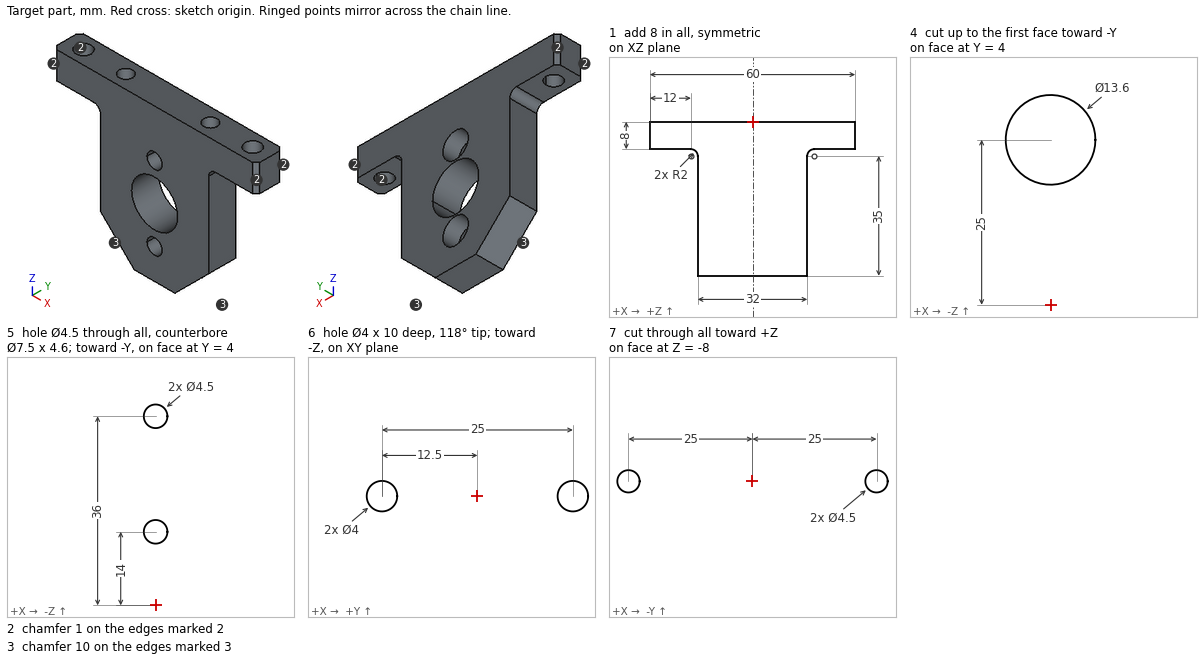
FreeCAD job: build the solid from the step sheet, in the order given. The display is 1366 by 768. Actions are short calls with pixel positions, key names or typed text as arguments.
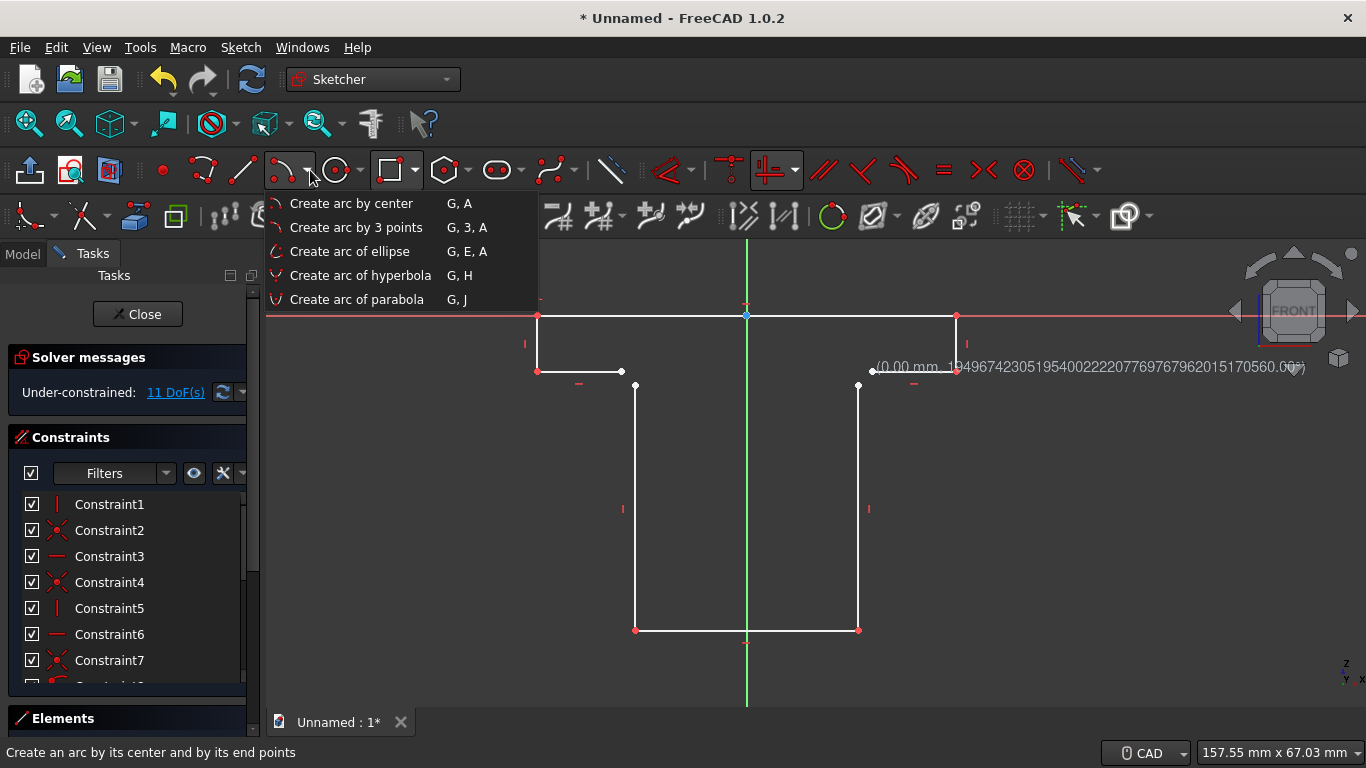
click(402, 227)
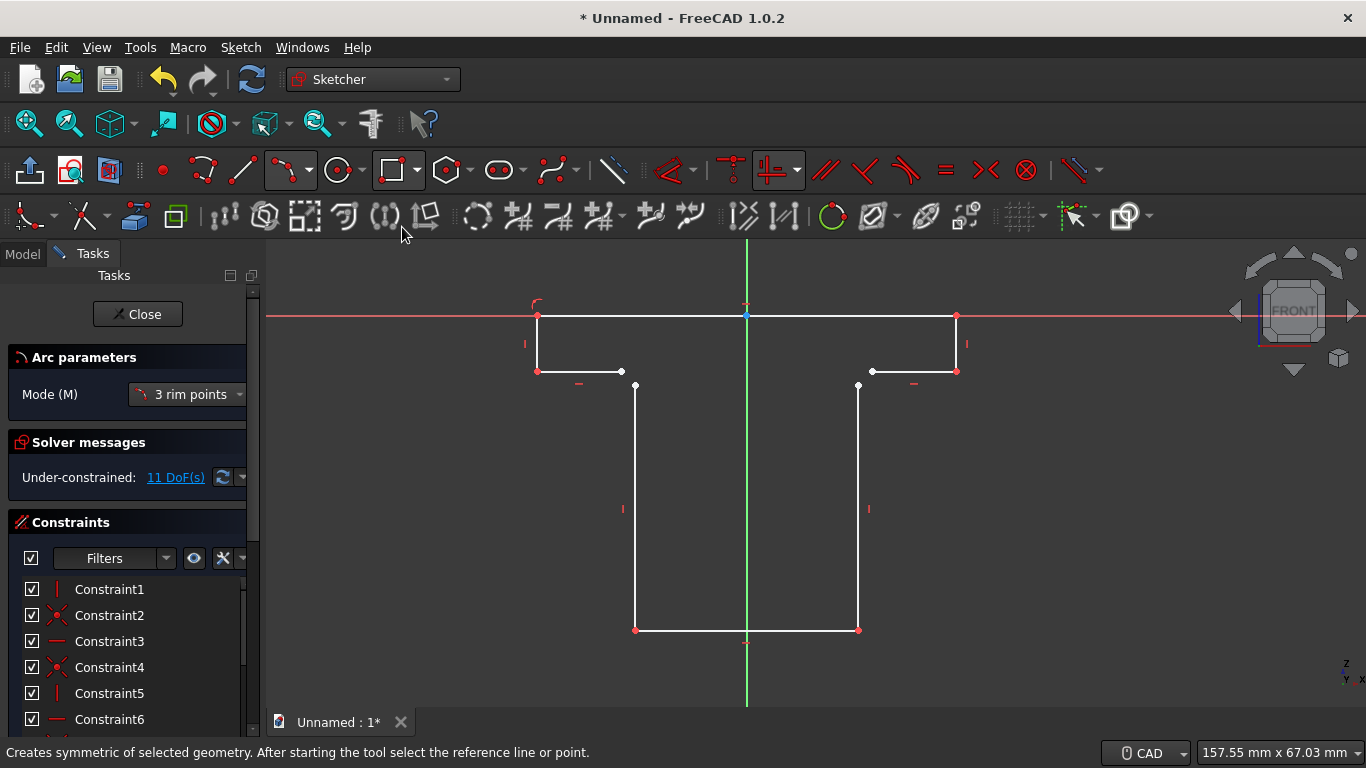
click(635, 386)
click(621, 372)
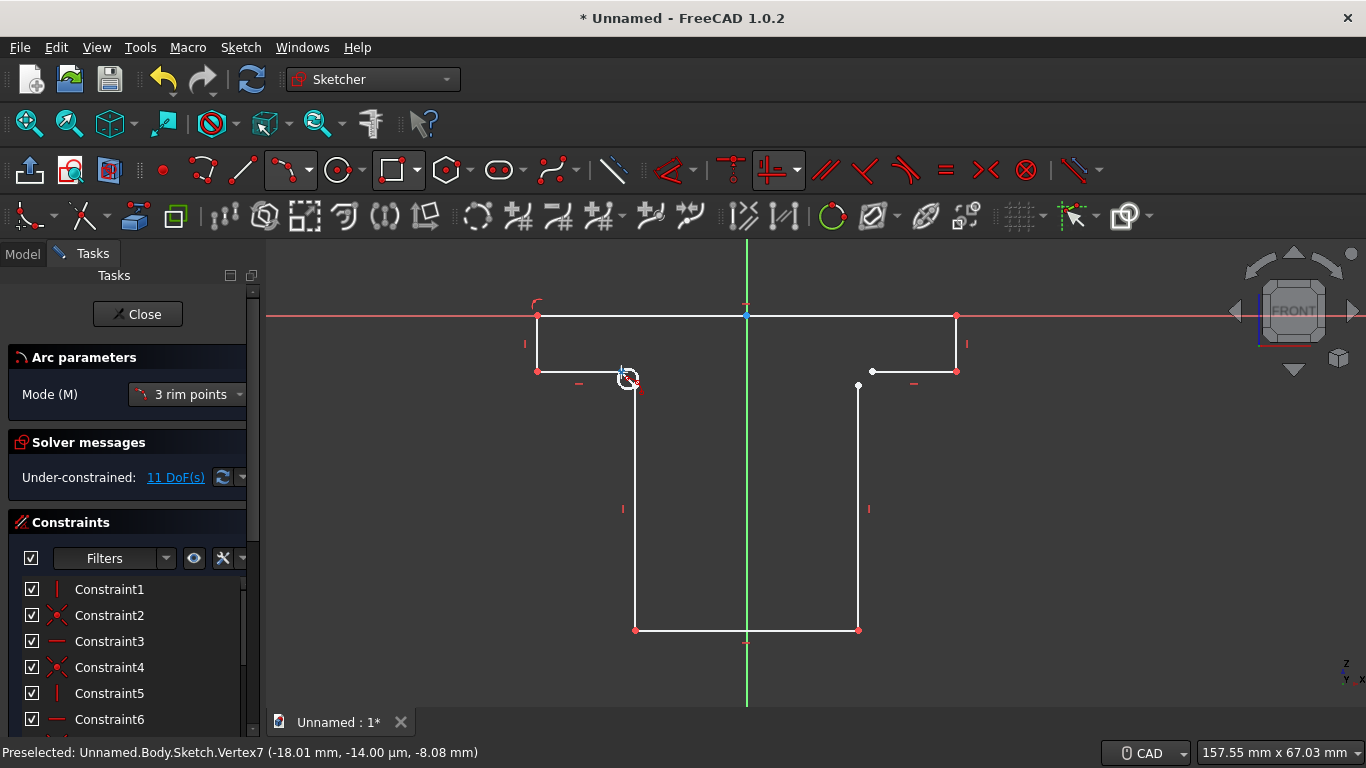
scroll(631, 376, up, 7)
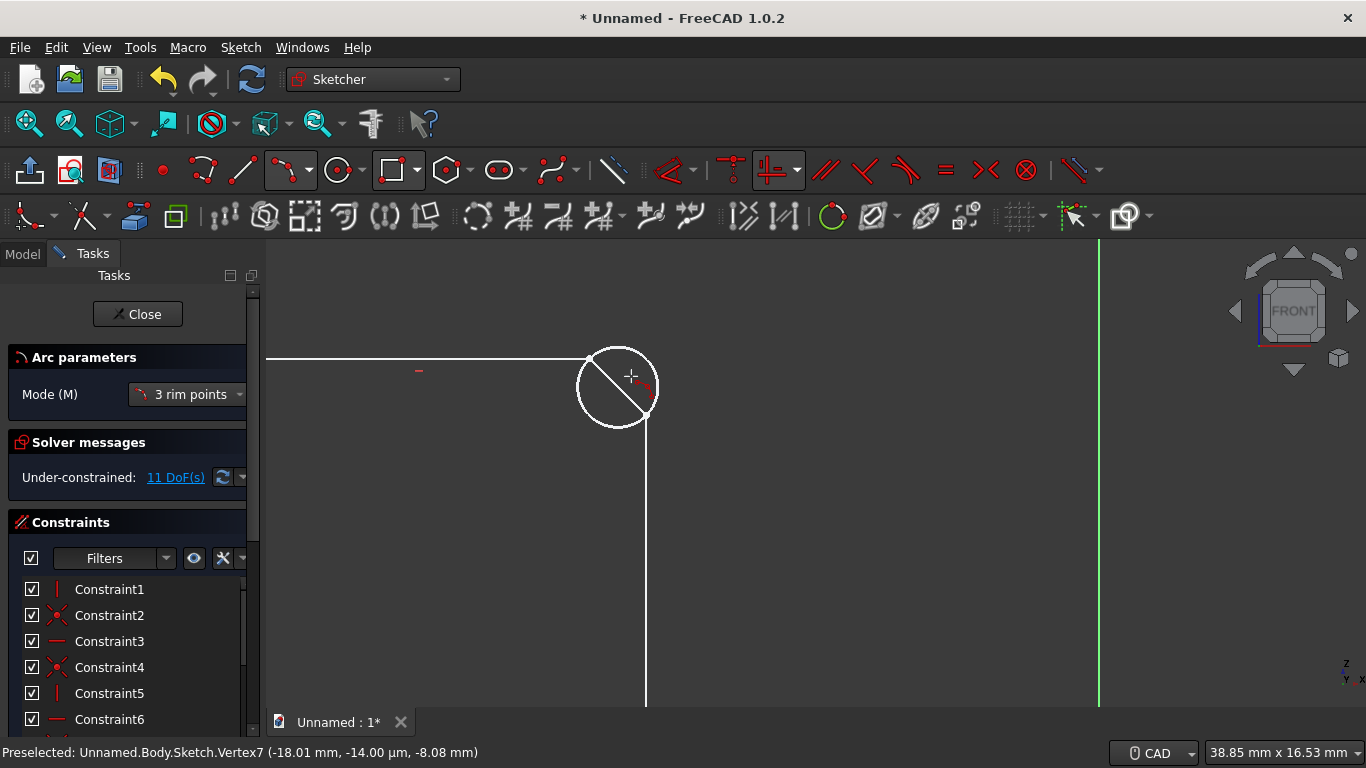
click(630, 373)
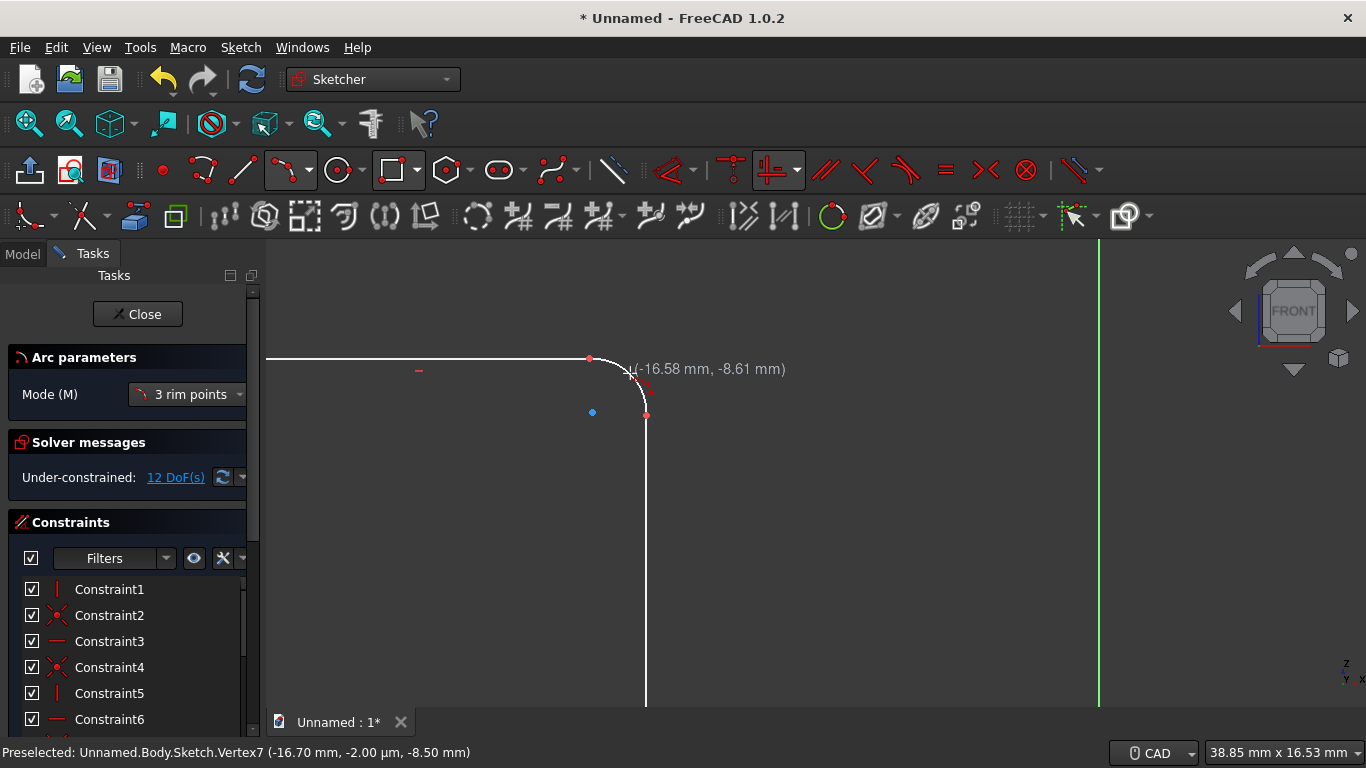
scroll(632, 377, down, 7)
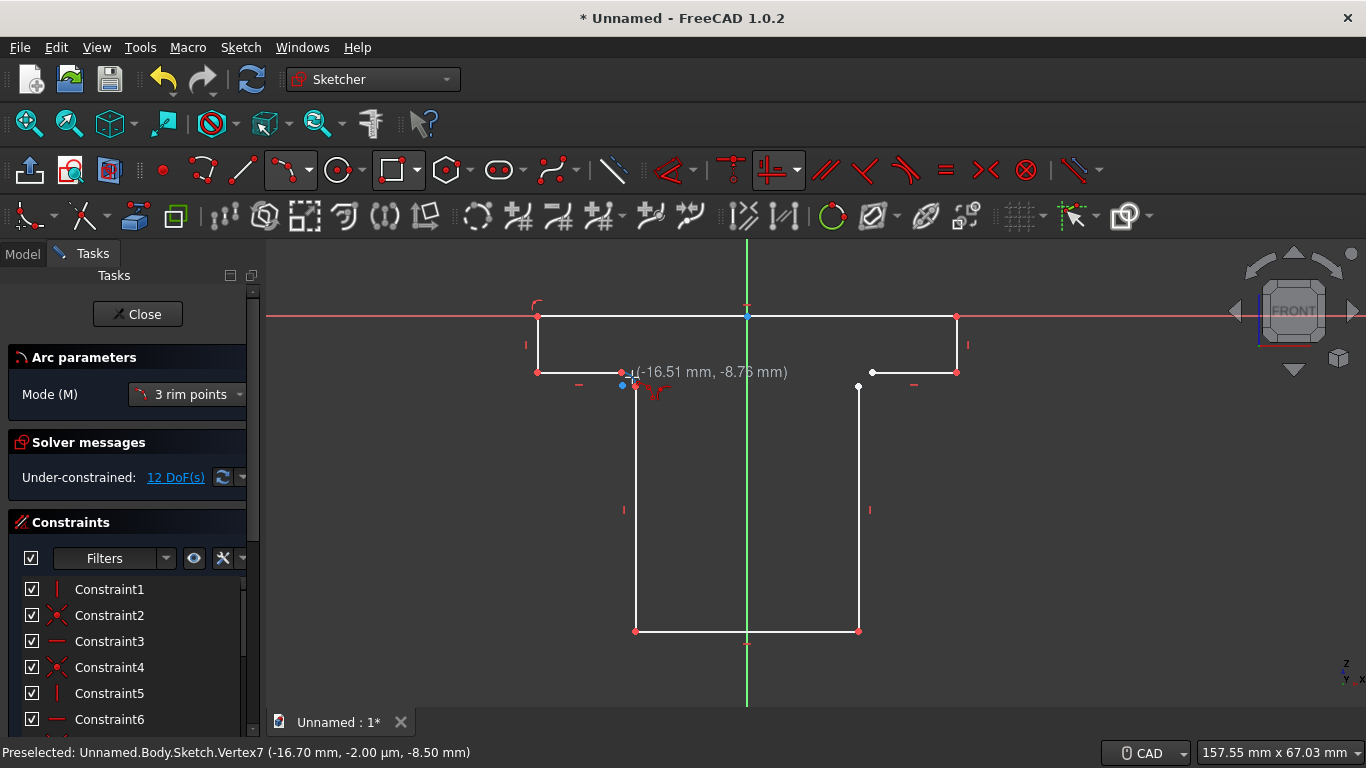
click(873, 373)
click(859, 387)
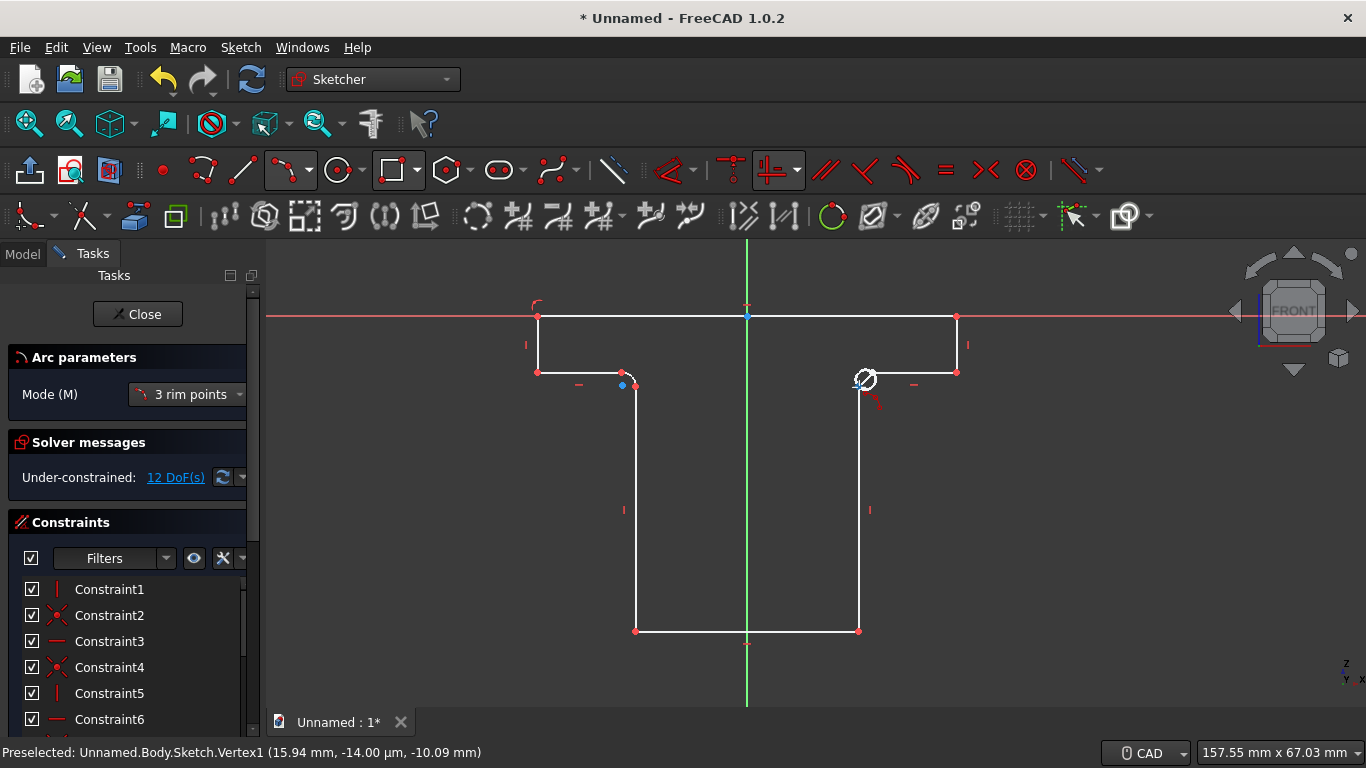
scroll(863, 376, up, 7)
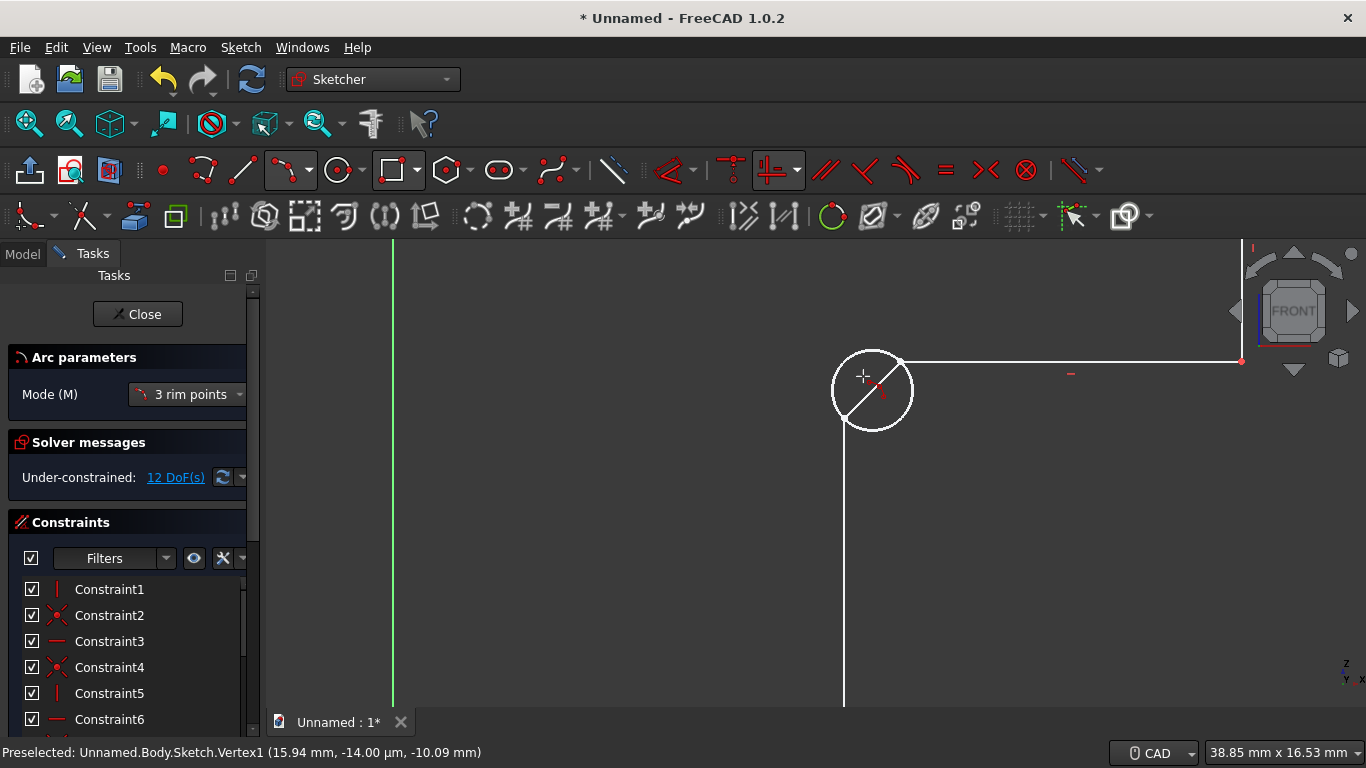
click(863, 376)
key(Escape)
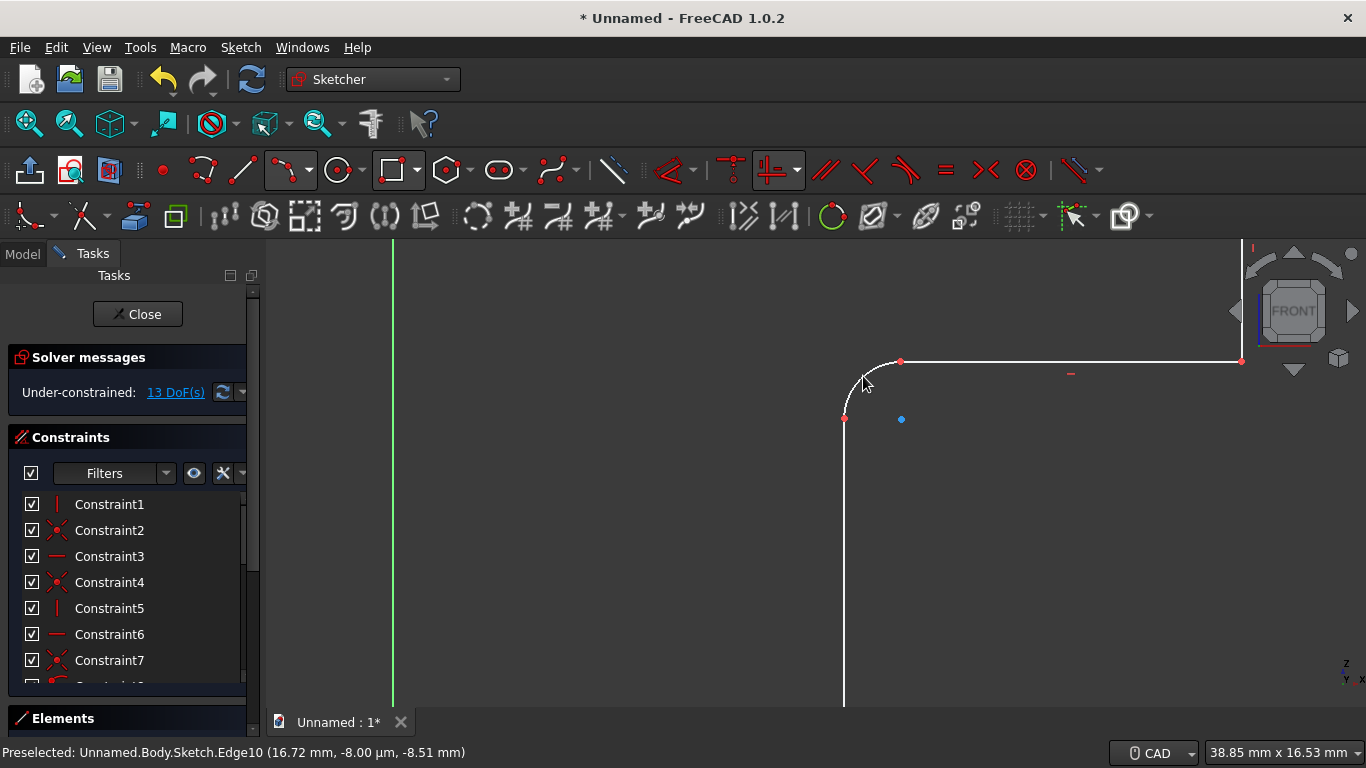
scroll(864, 376, down, 7)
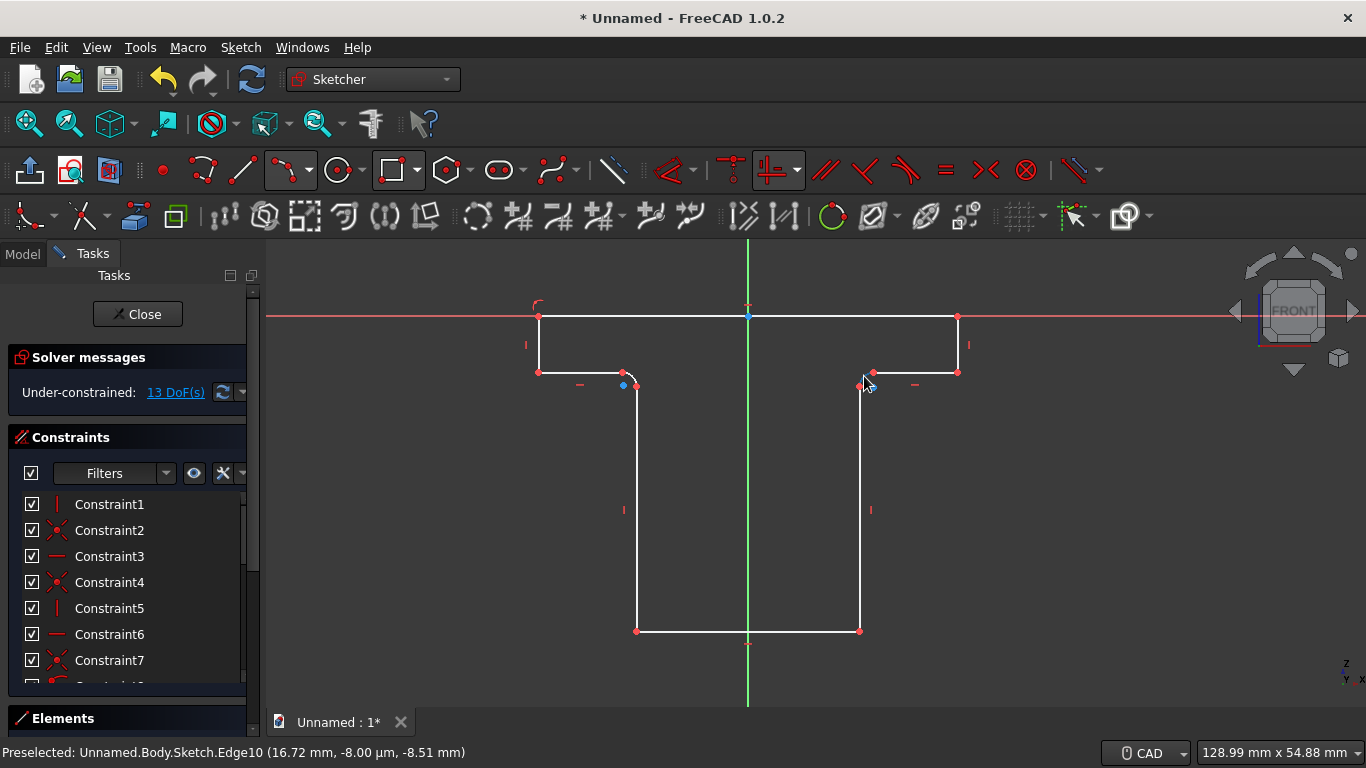
click(860, 436)